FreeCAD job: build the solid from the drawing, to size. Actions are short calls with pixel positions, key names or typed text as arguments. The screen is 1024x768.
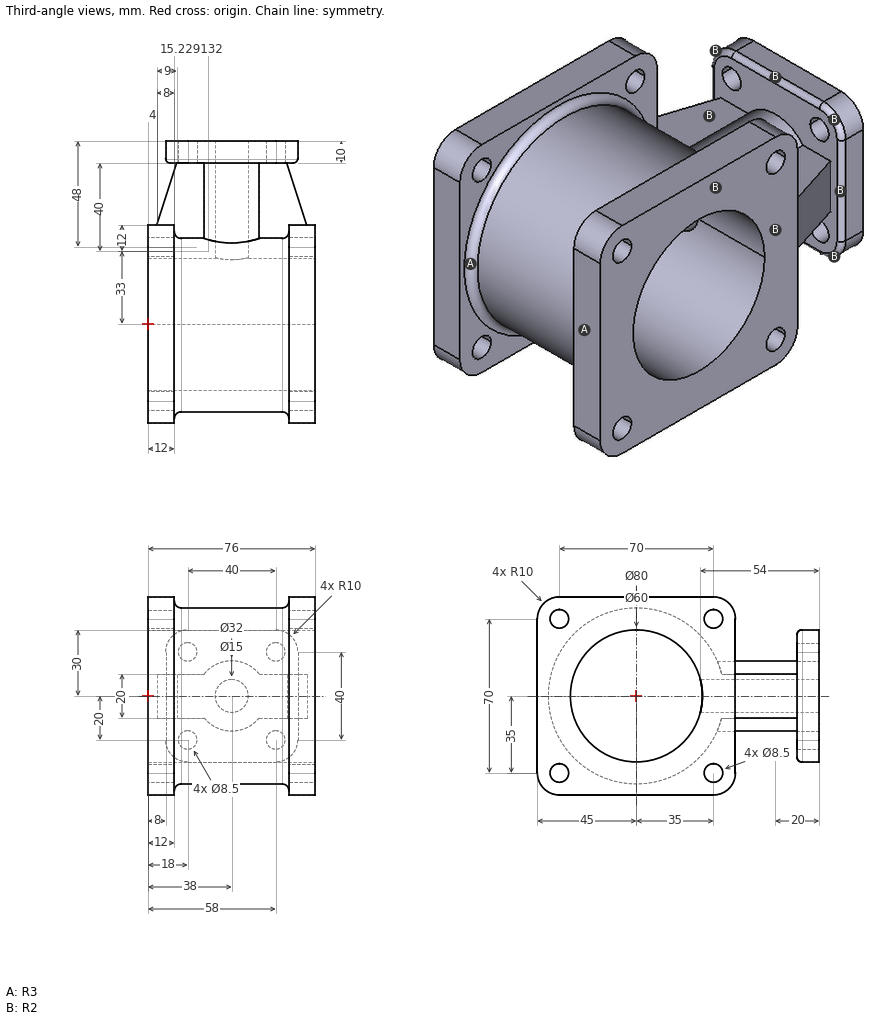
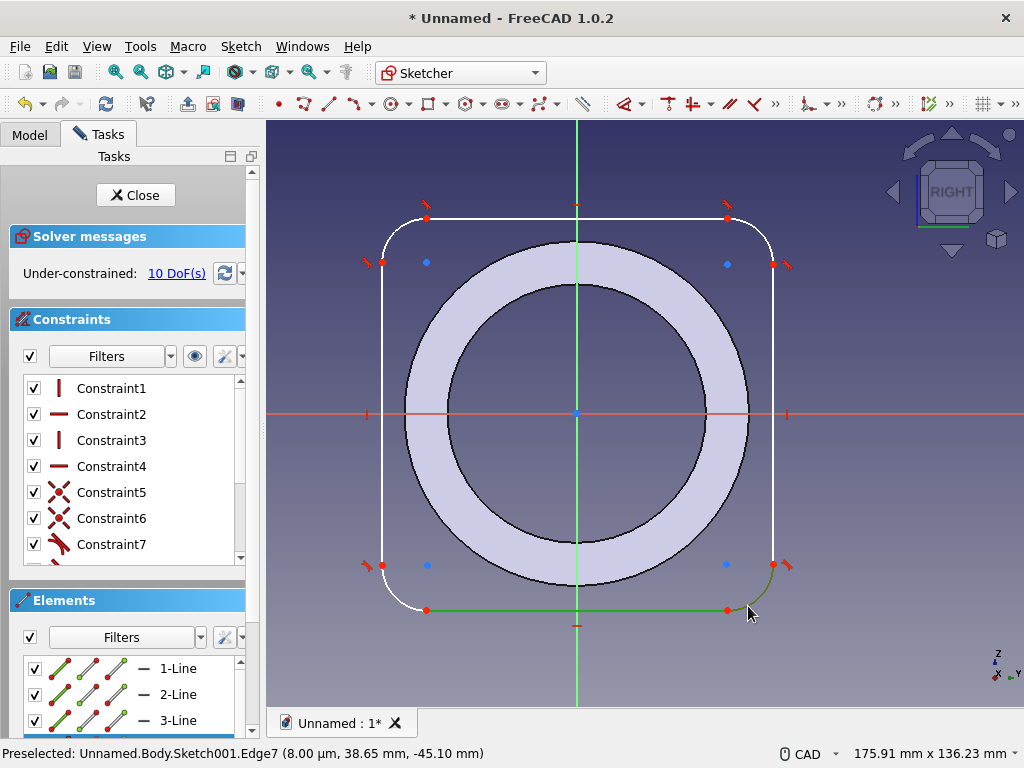
key(t)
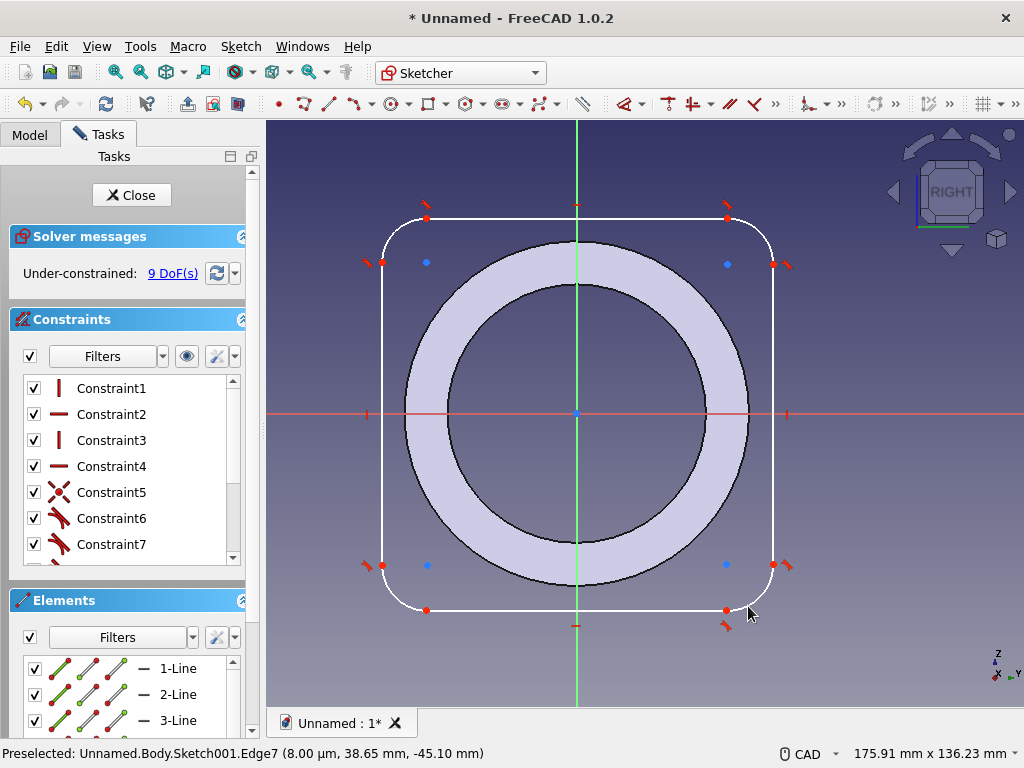
click(637, 611)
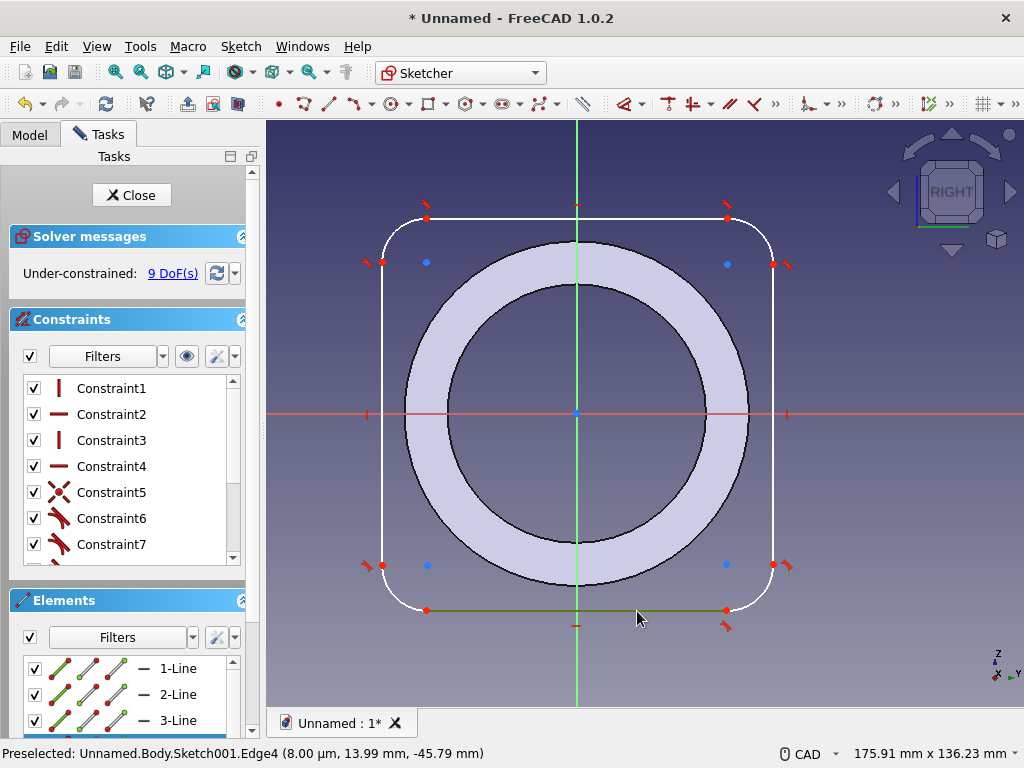
click(387, 586)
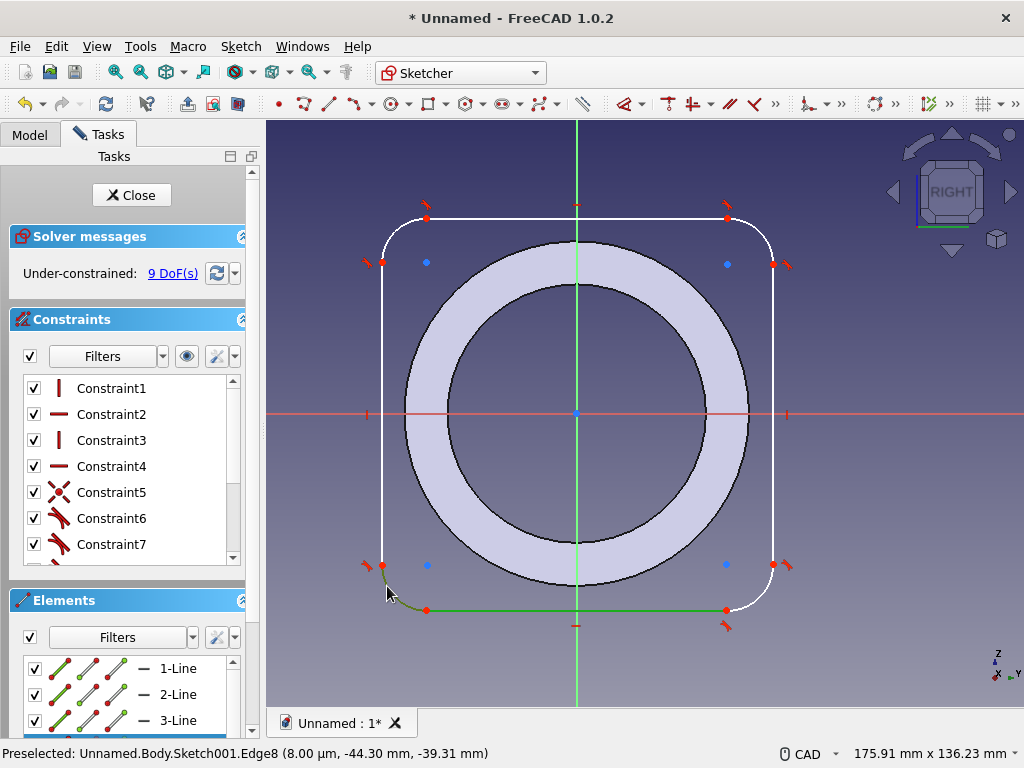
key(t)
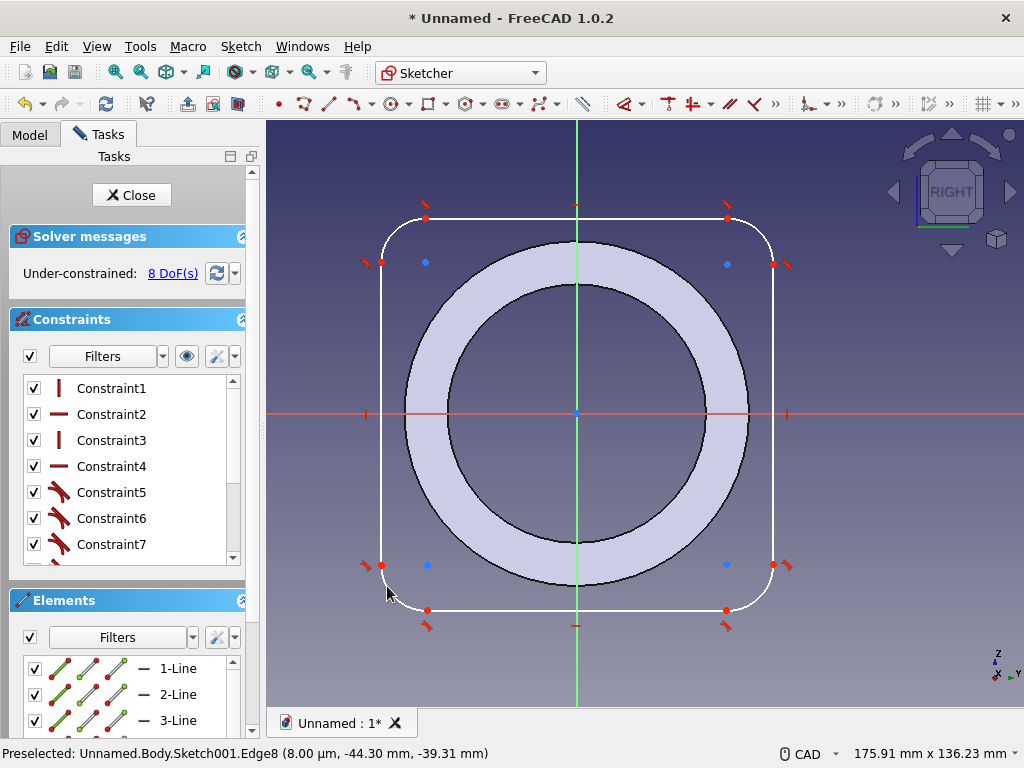
click(405, 224)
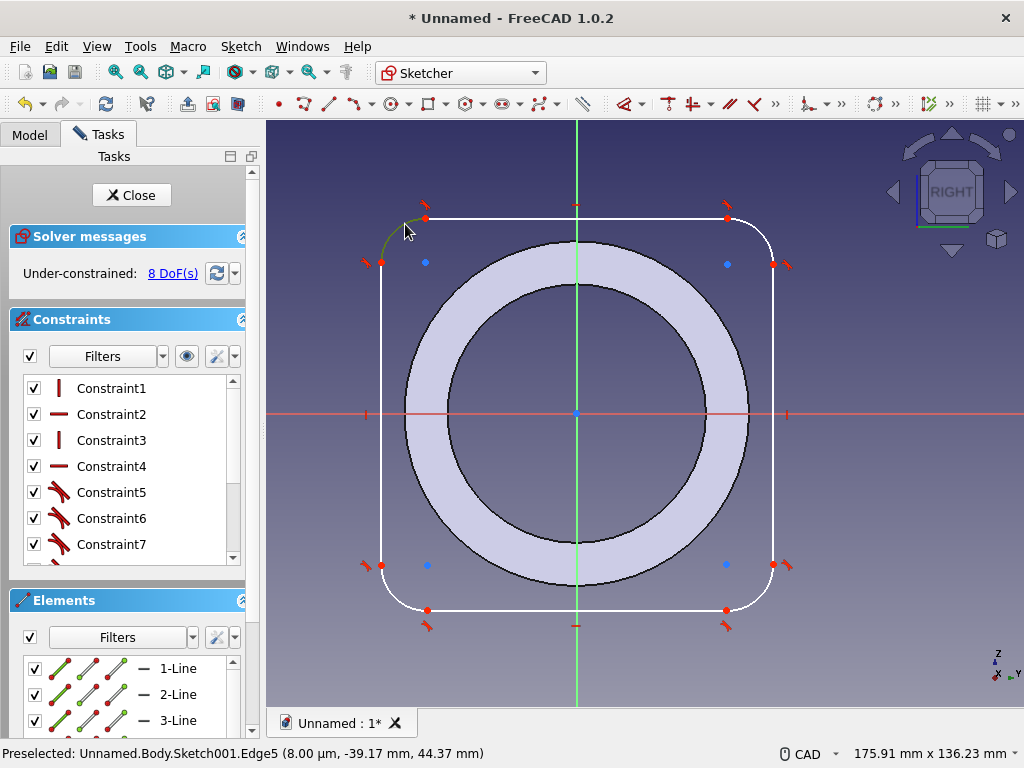
click(768, 244)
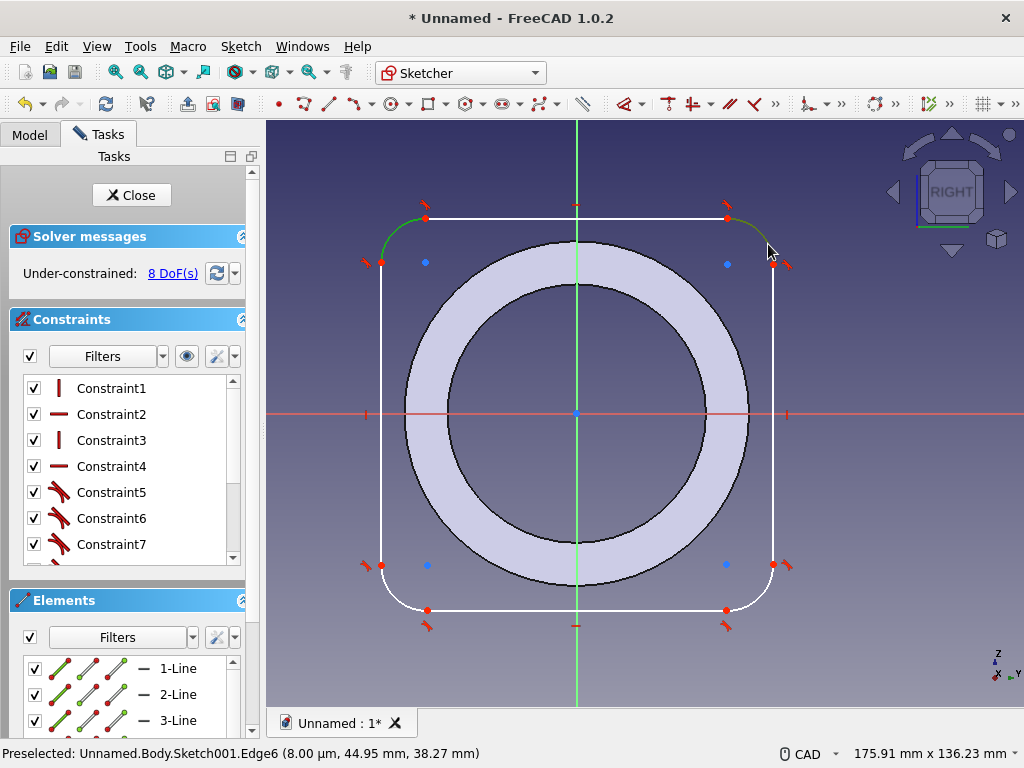
click(748, 606)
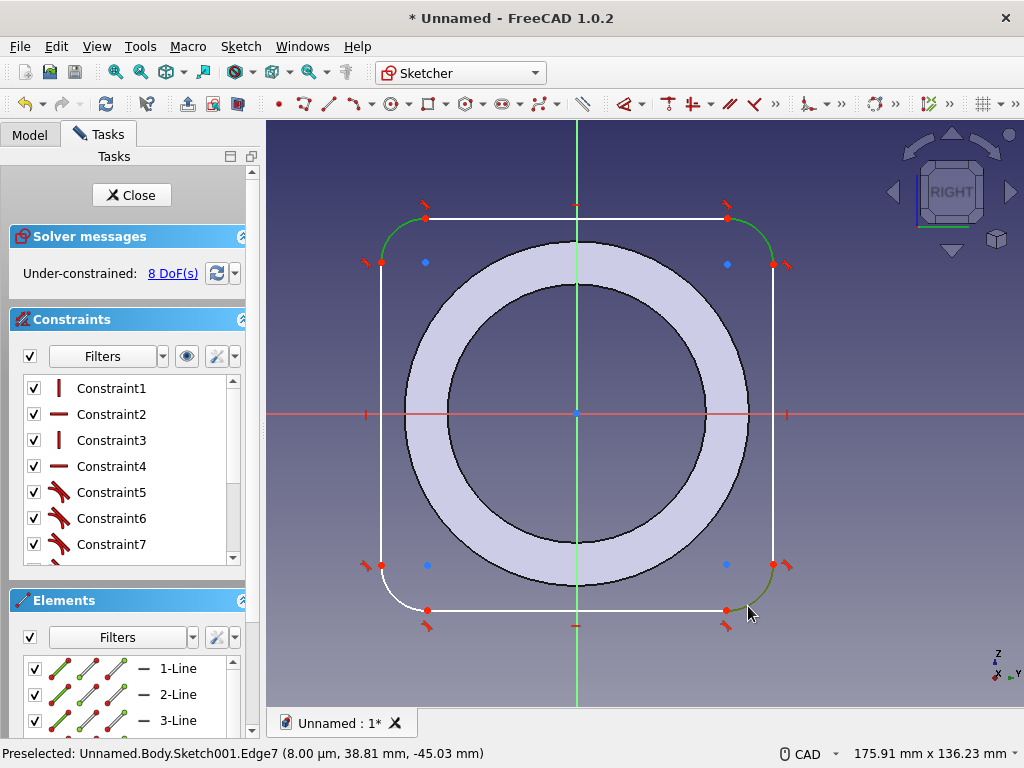
click(386, 586)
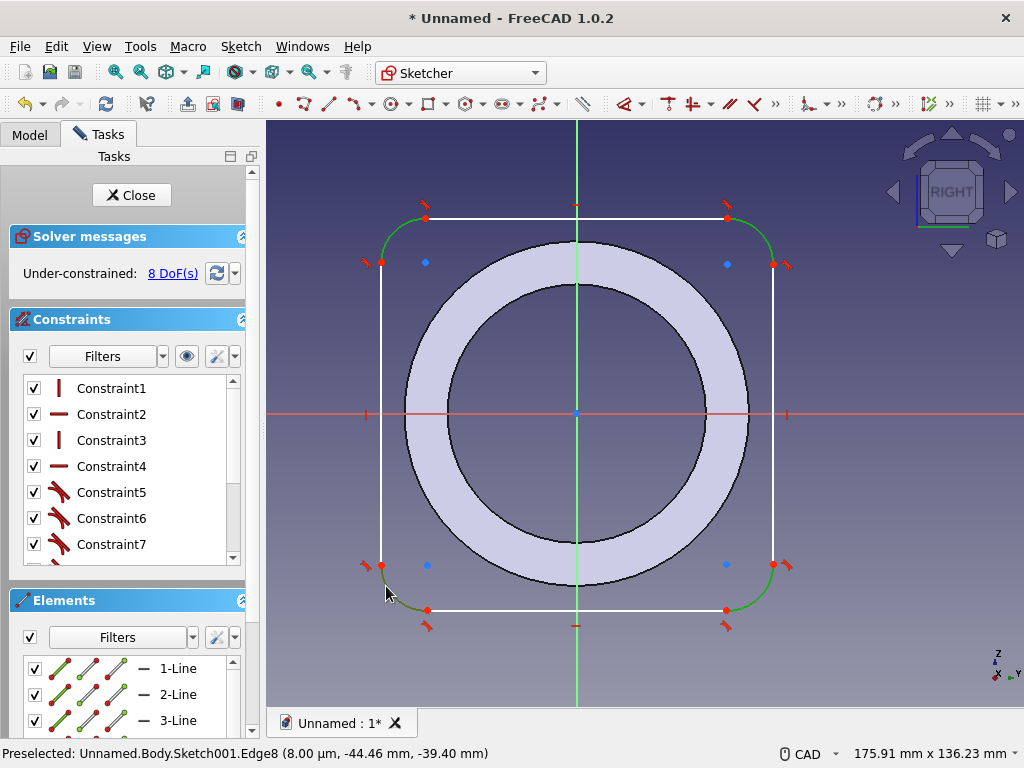
key(e)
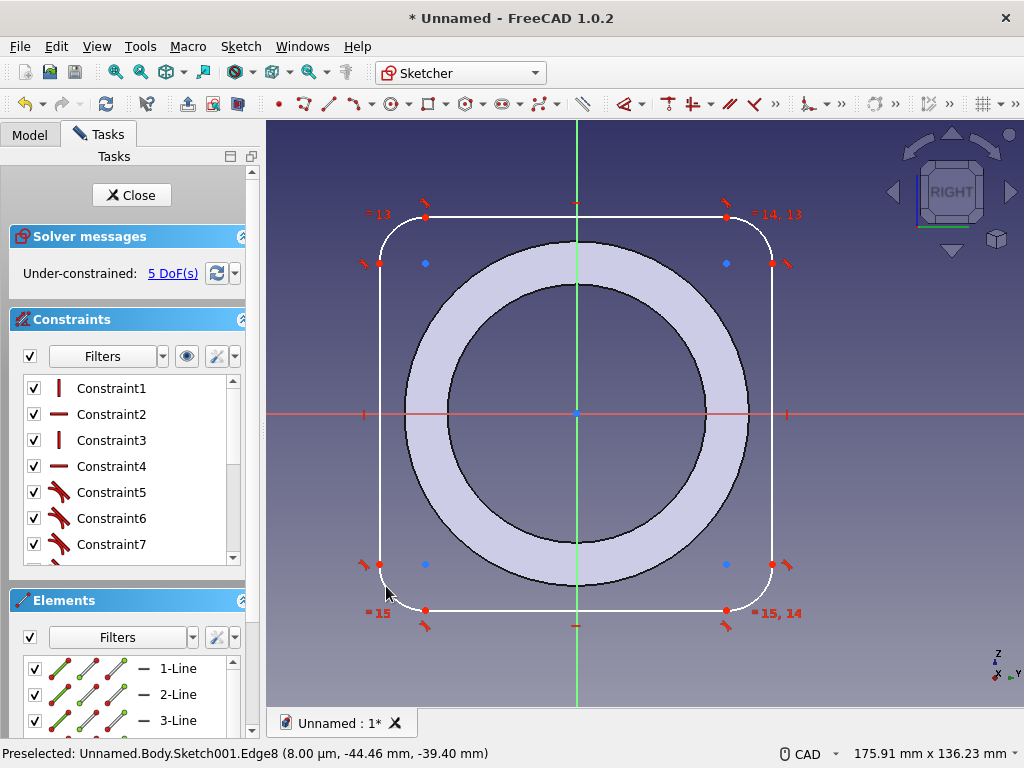
click(624, 104)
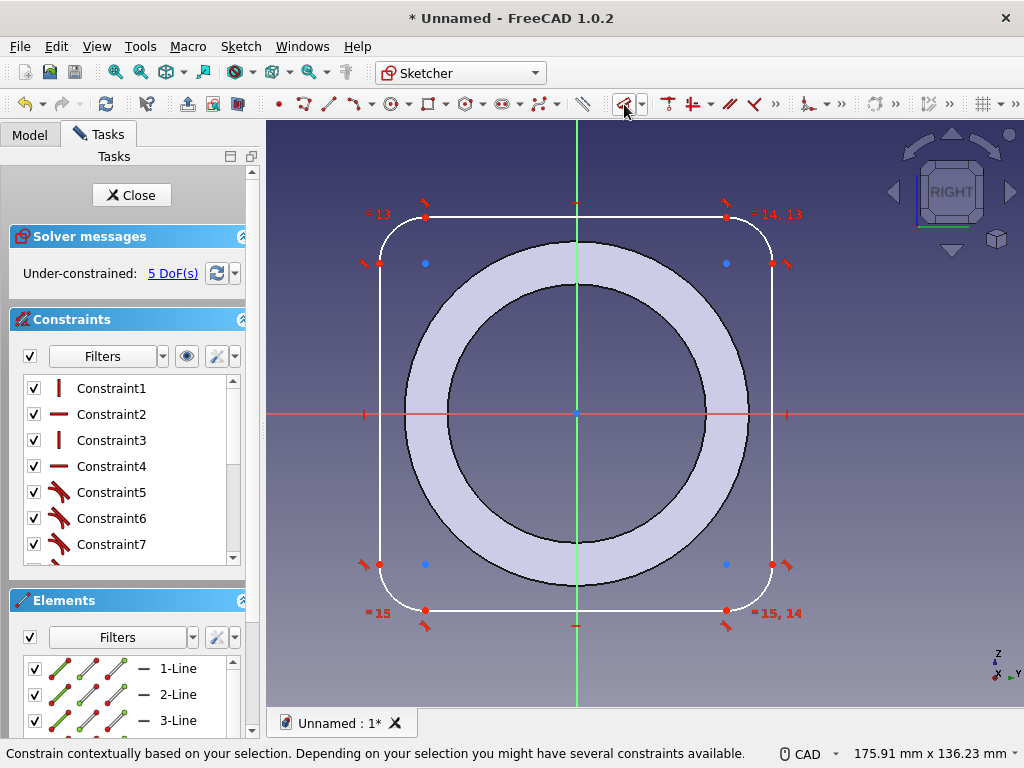
click(405, 222)
click(391, 193)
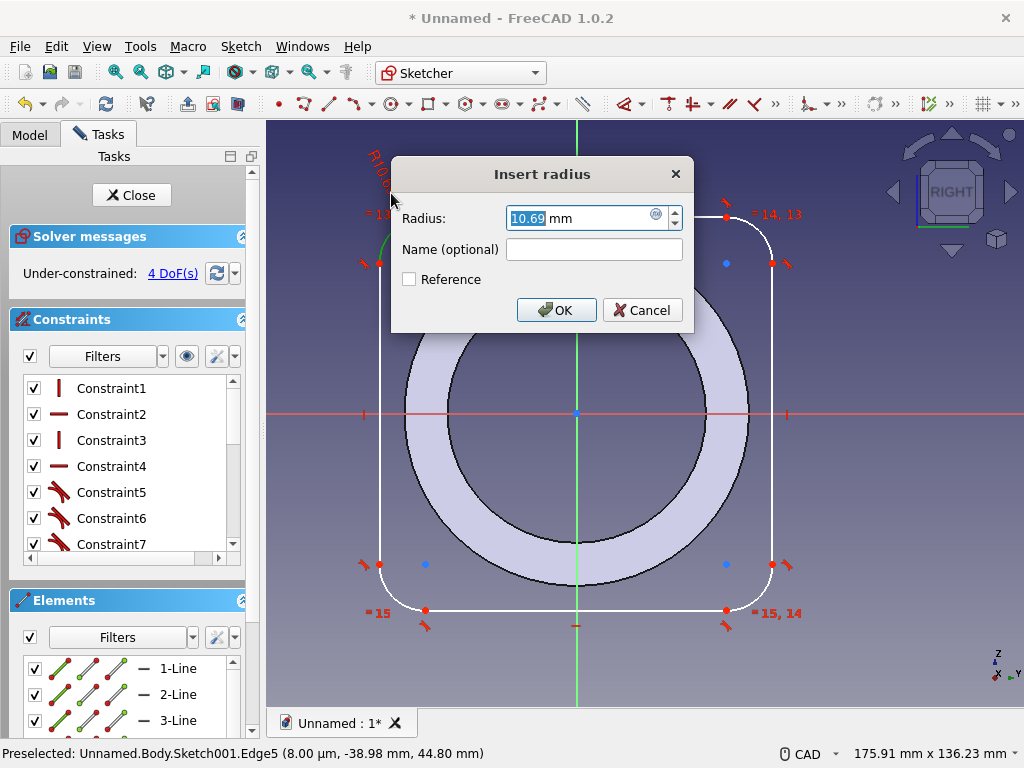
text(10)
key(Return)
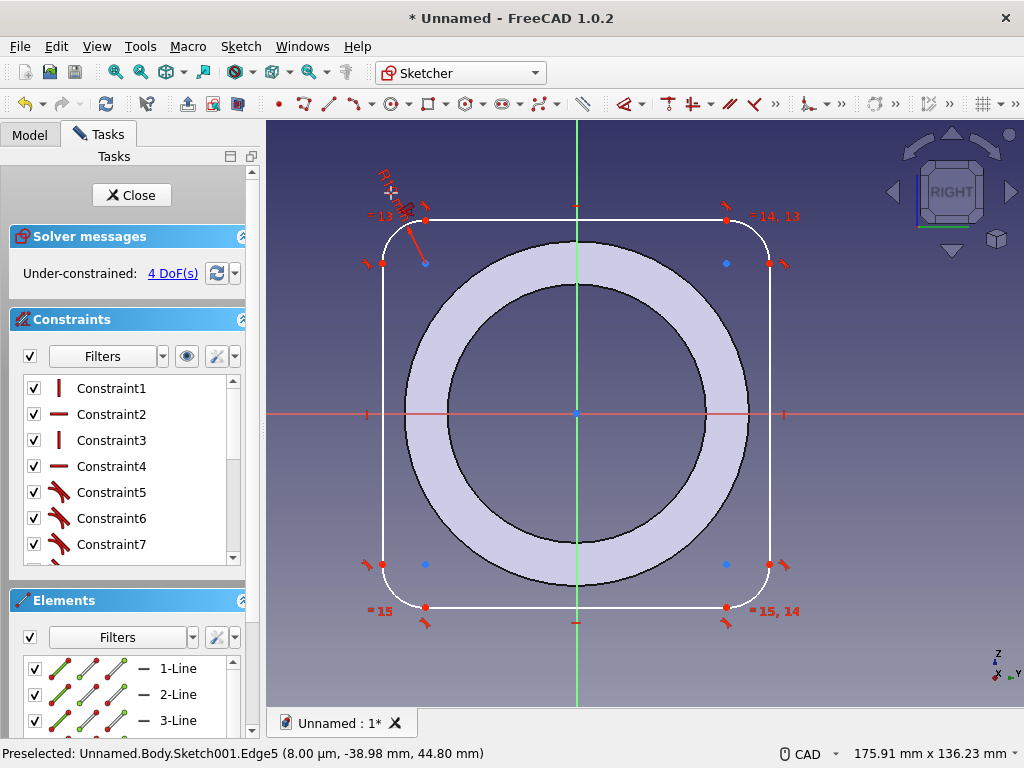
click(383, 474)
click(349, 345)